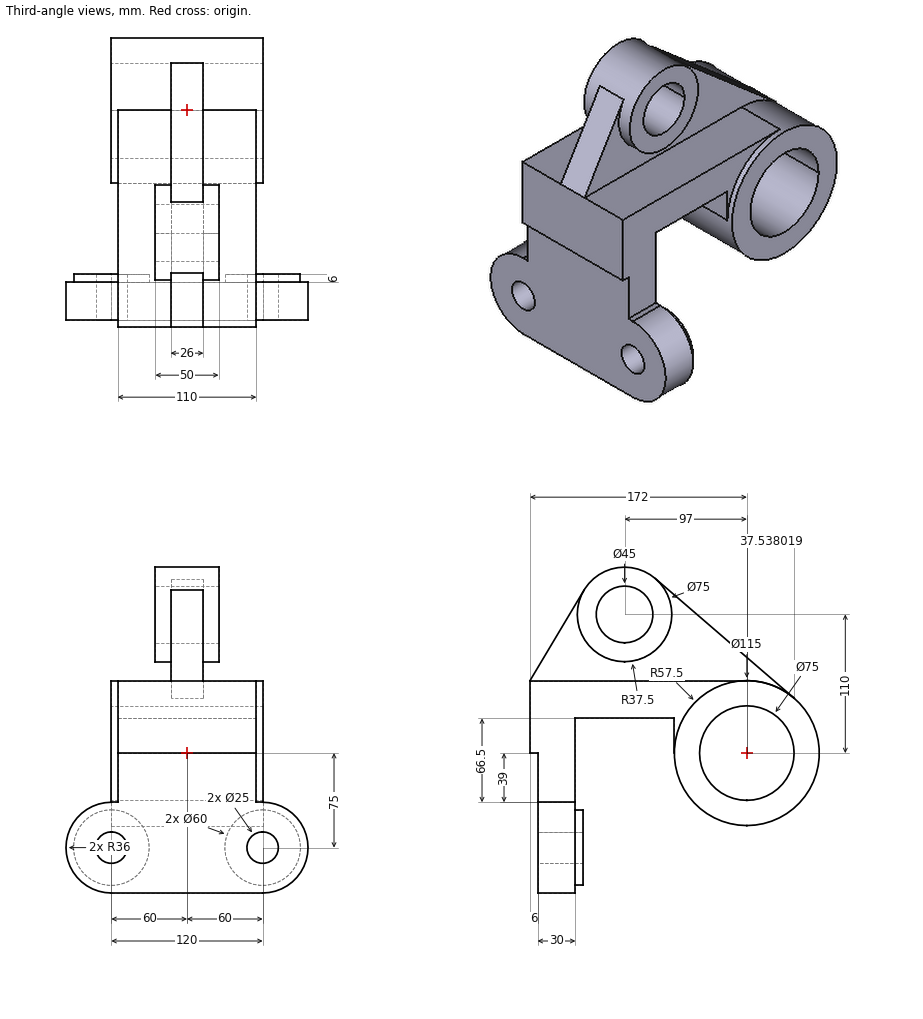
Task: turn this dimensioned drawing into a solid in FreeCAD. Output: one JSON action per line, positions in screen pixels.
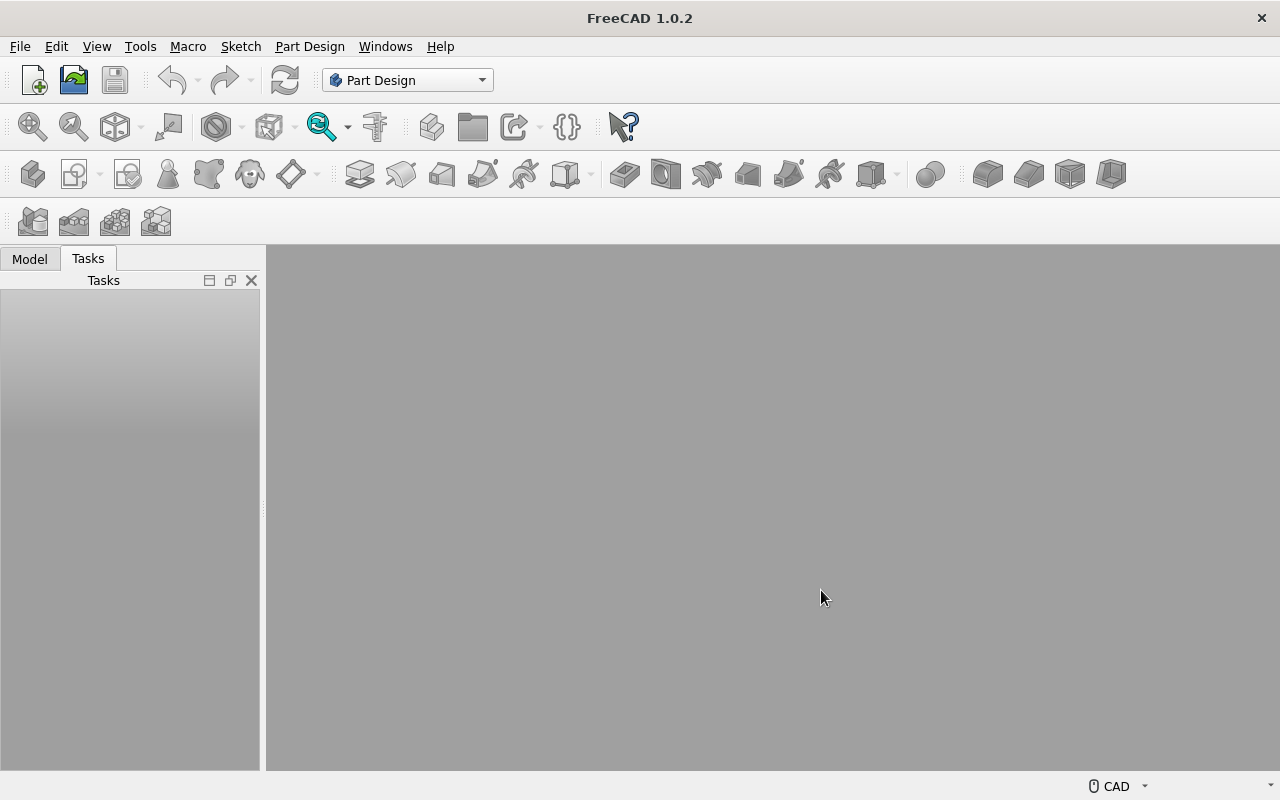
{"action": "left_click", "coordinate": [33, 80]}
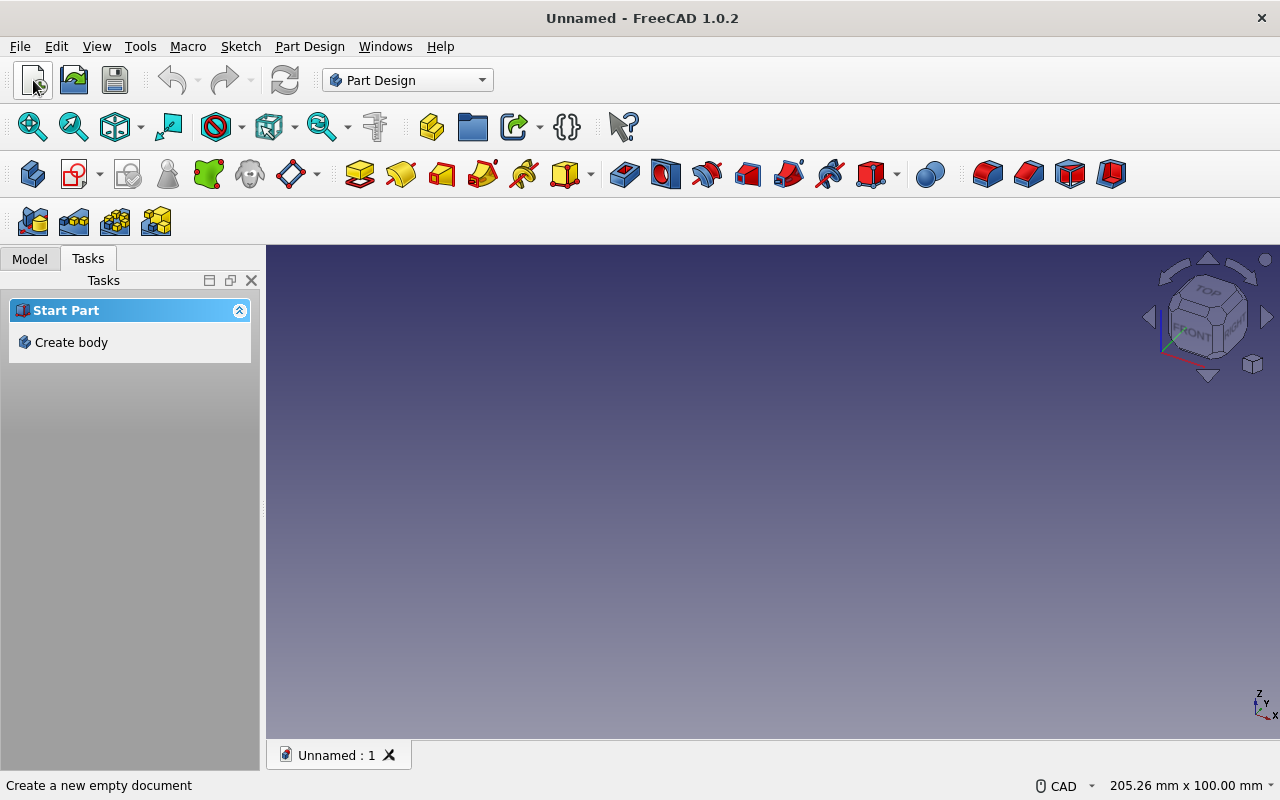
{"action": "left_click", "coordinate": [74, 174]}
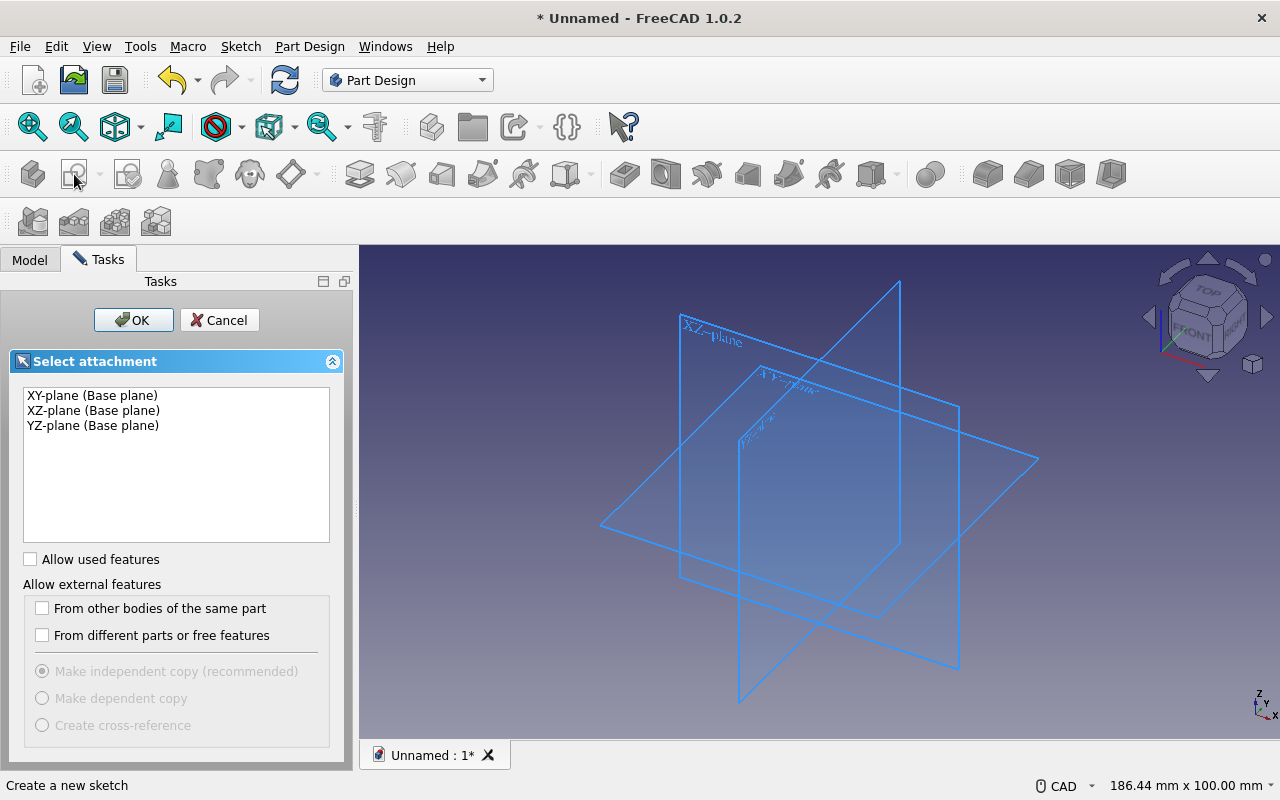
{"action": "left_click", "coordinate": [84, 426]}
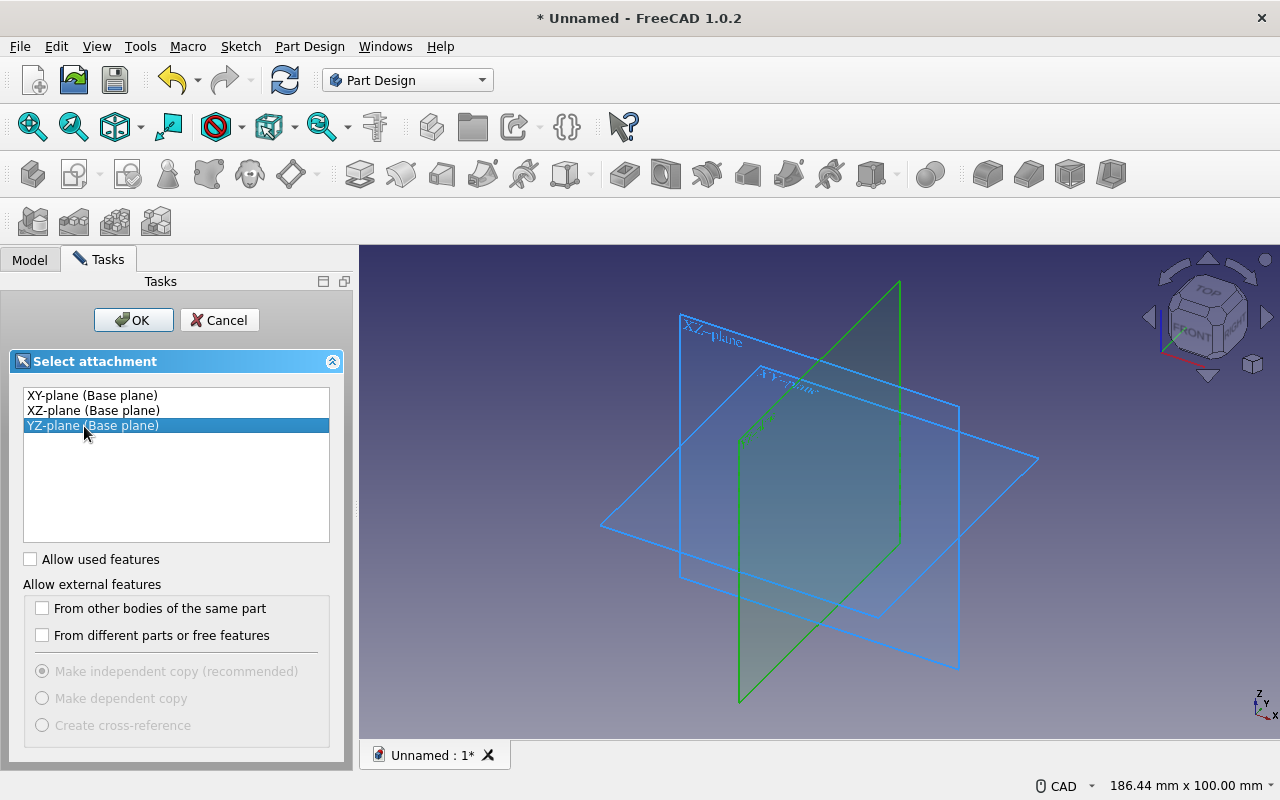
{"action": "left_click", "coordinate": [134, 320]}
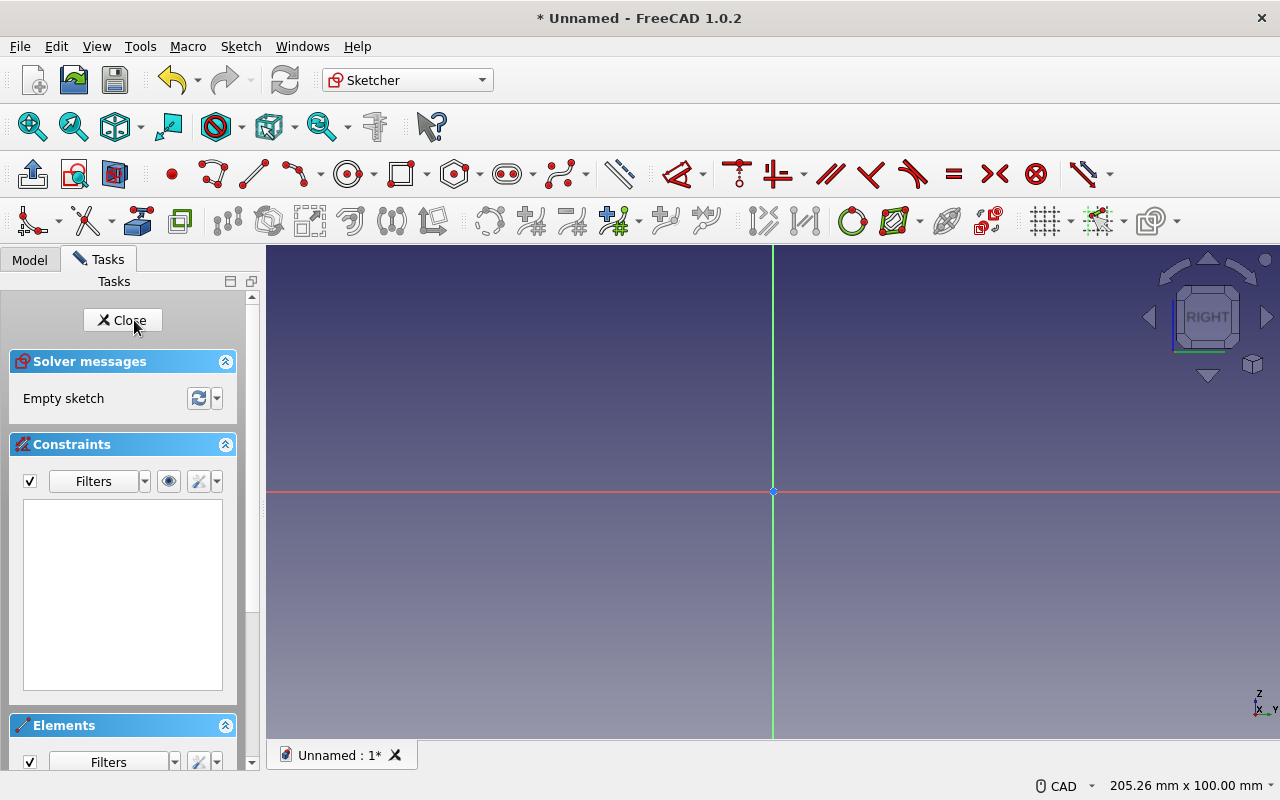
{"action": "scroll", "coordinate": [621, 492], "scroll_direction": "down", "scroll_amount": 3}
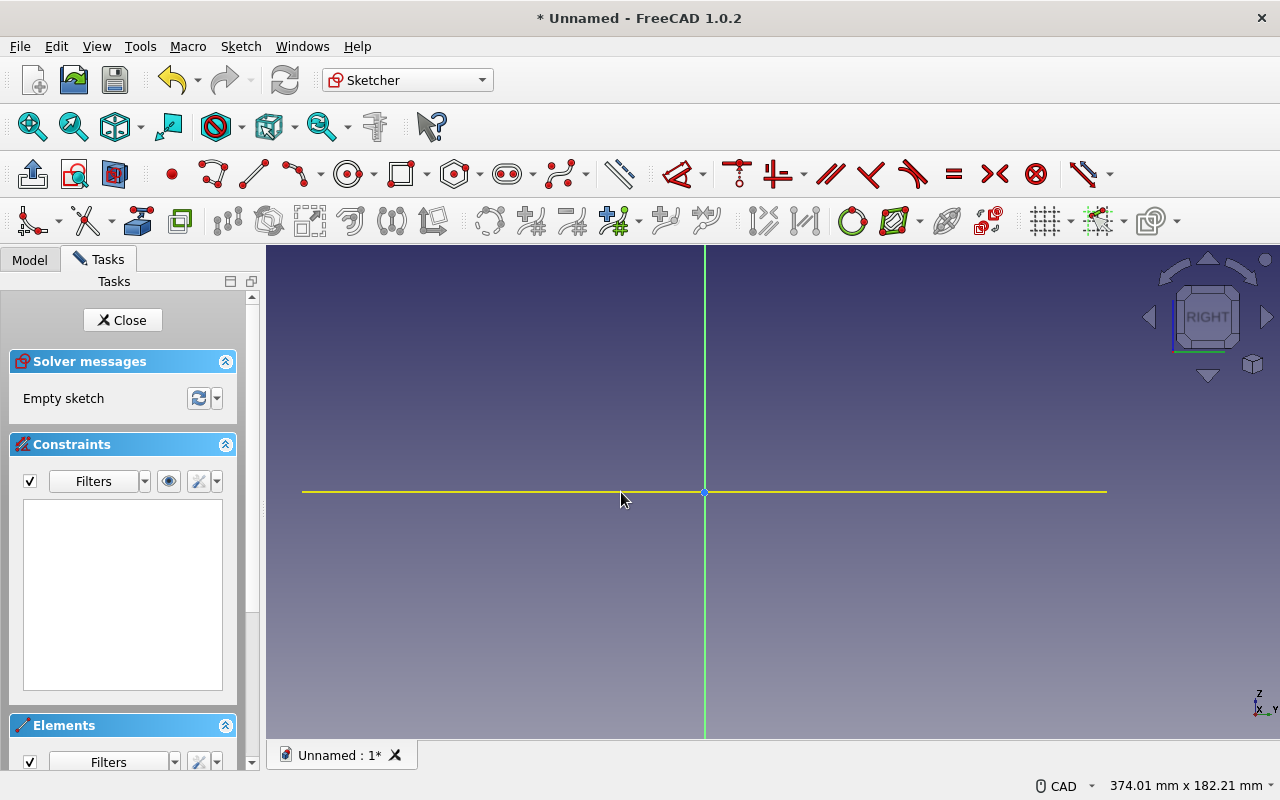
{"action": "key", "text": "g c"}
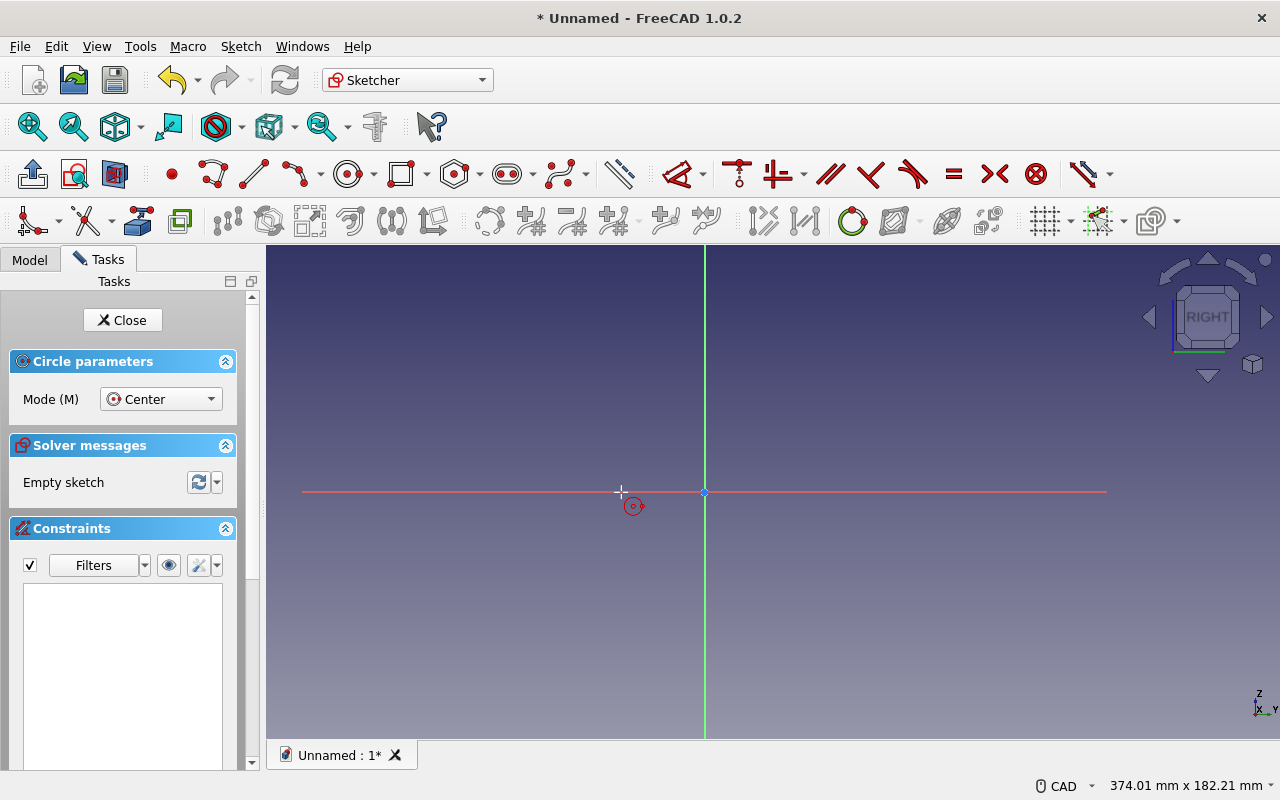
{"action": "left_click", "coordinate": [705, 492]}
{"action": "left_click", "coordinate": [815, 382]}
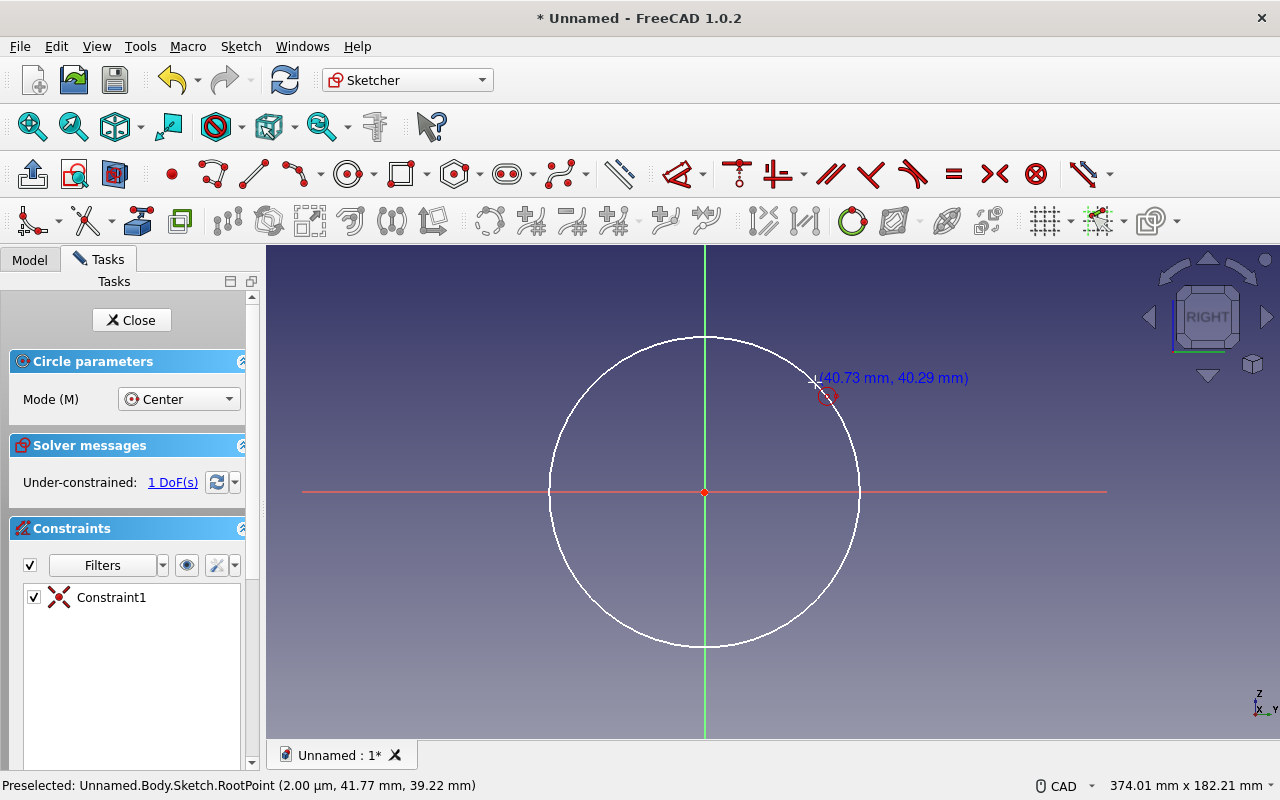
{"action": "left_click", "coordinate": [705, 492]}
{"action": "left_click", "coordinate": [776, 420]}
{"action": "key", "text": "Escape"}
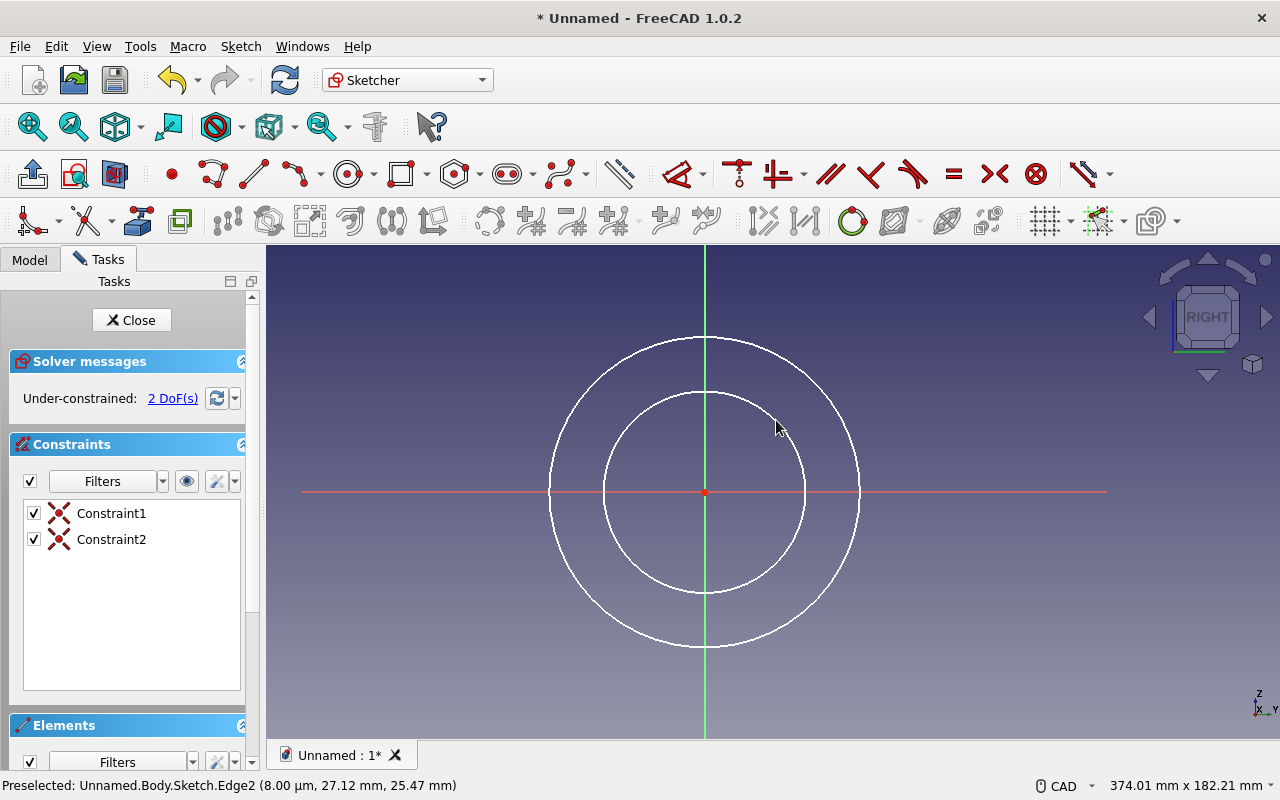
{"action": "left_click", "coordinate": [676, 174]}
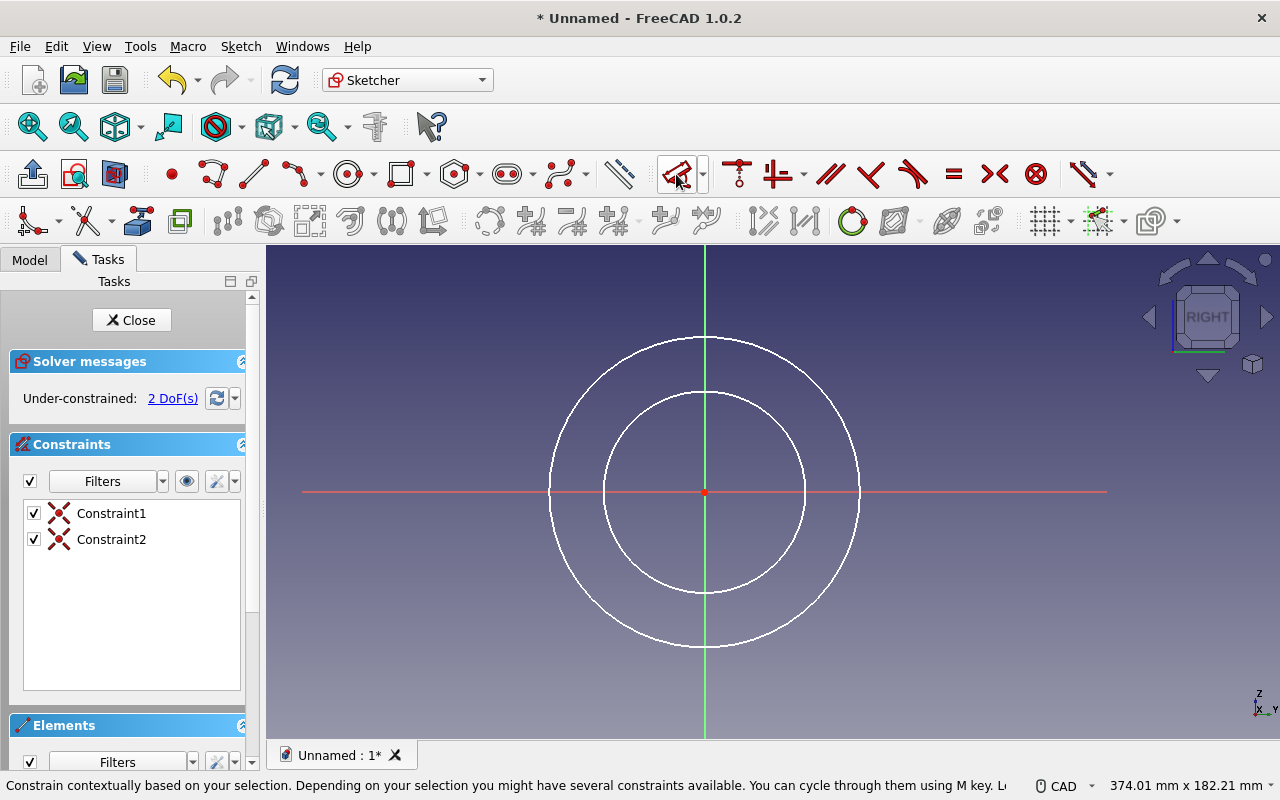
{"action": "left_click", "coordinate": [814, 382]}
{"action": "left_click", "coordinate": [837, 359]}